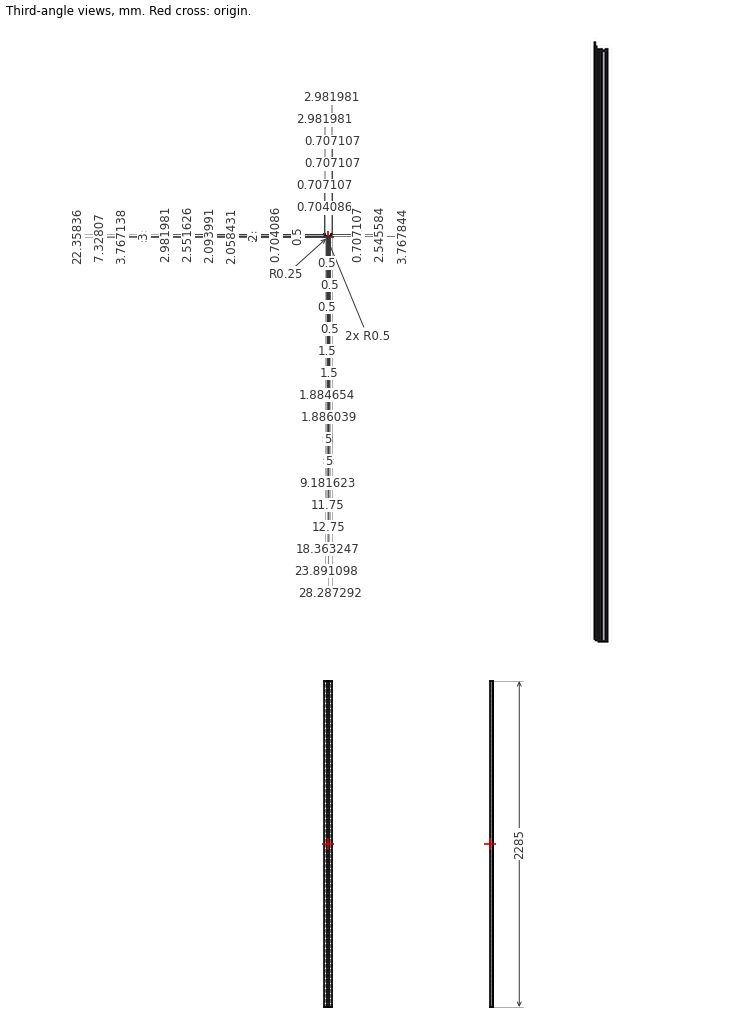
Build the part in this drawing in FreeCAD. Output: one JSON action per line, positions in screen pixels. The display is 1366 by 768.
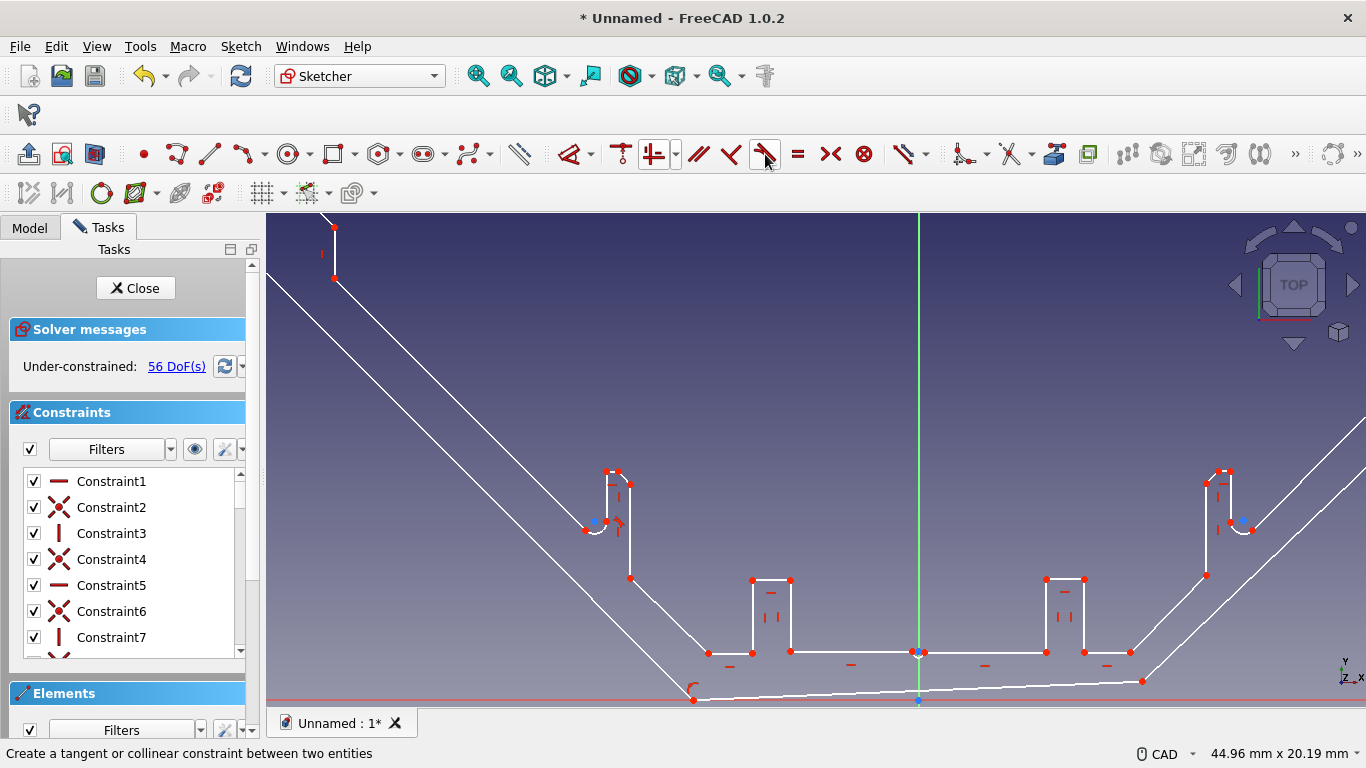
{"action": "left_click", "coordinate": [511, 455]}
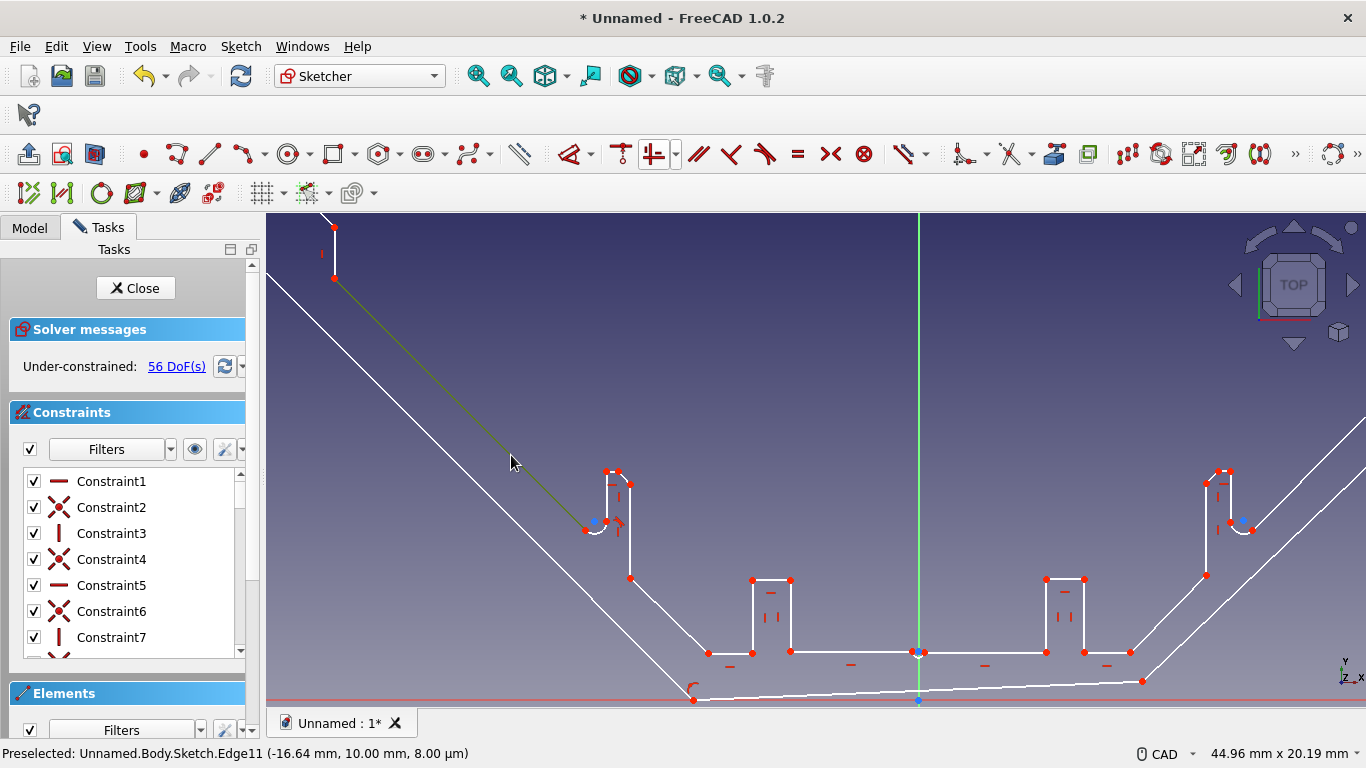
{"action": "left_click", "coordinate": [599, 533]}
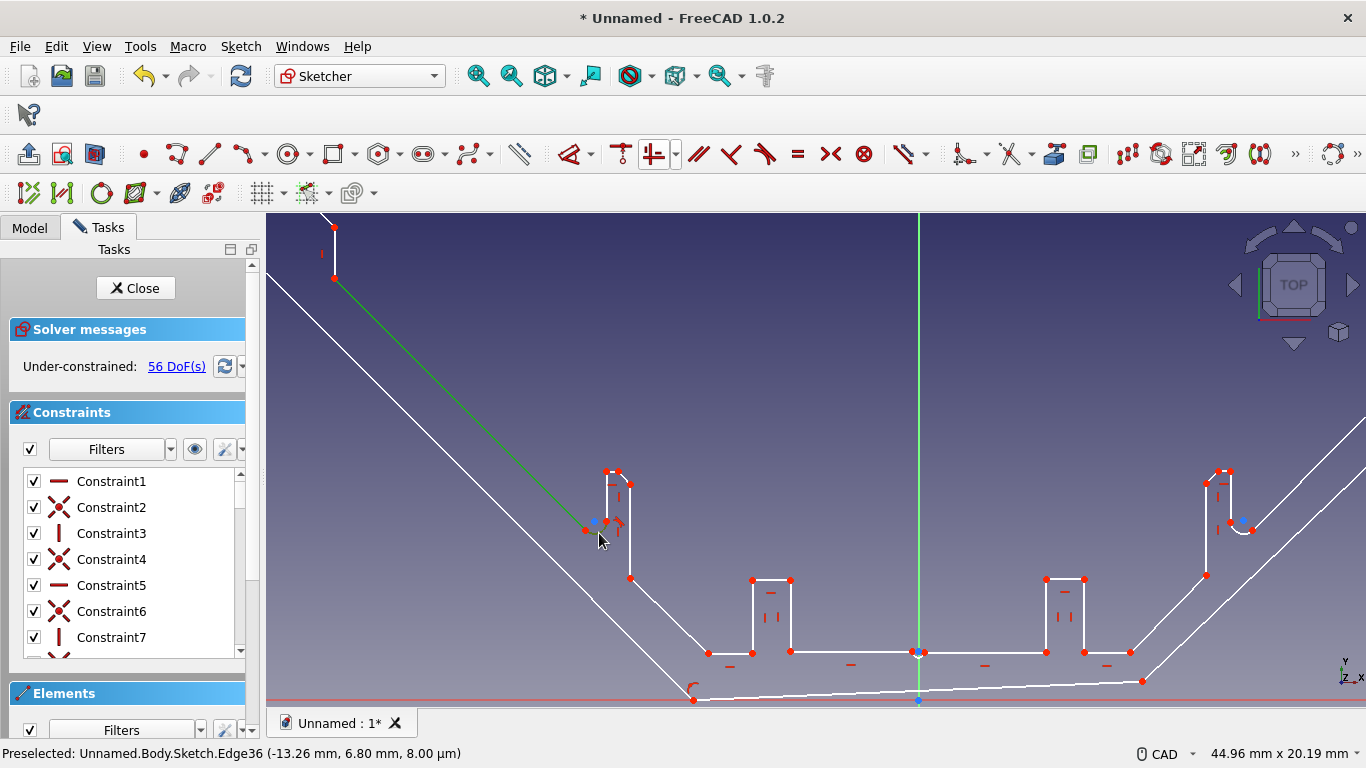
{"action": "left_click", "coordinate": [765, 154]}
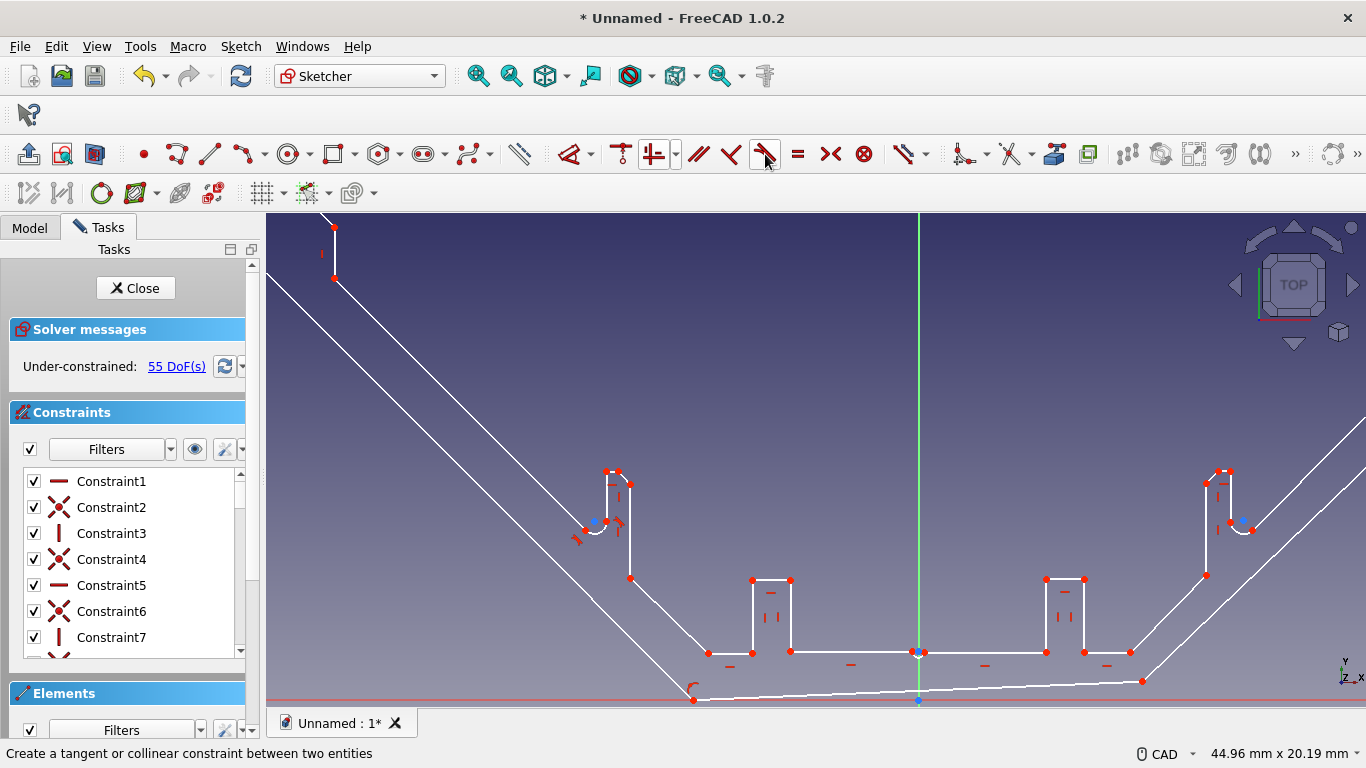
{"action": "scroll", "coordinate": [608, 487], "scroll_direction": "down", "scroll_amount": 4}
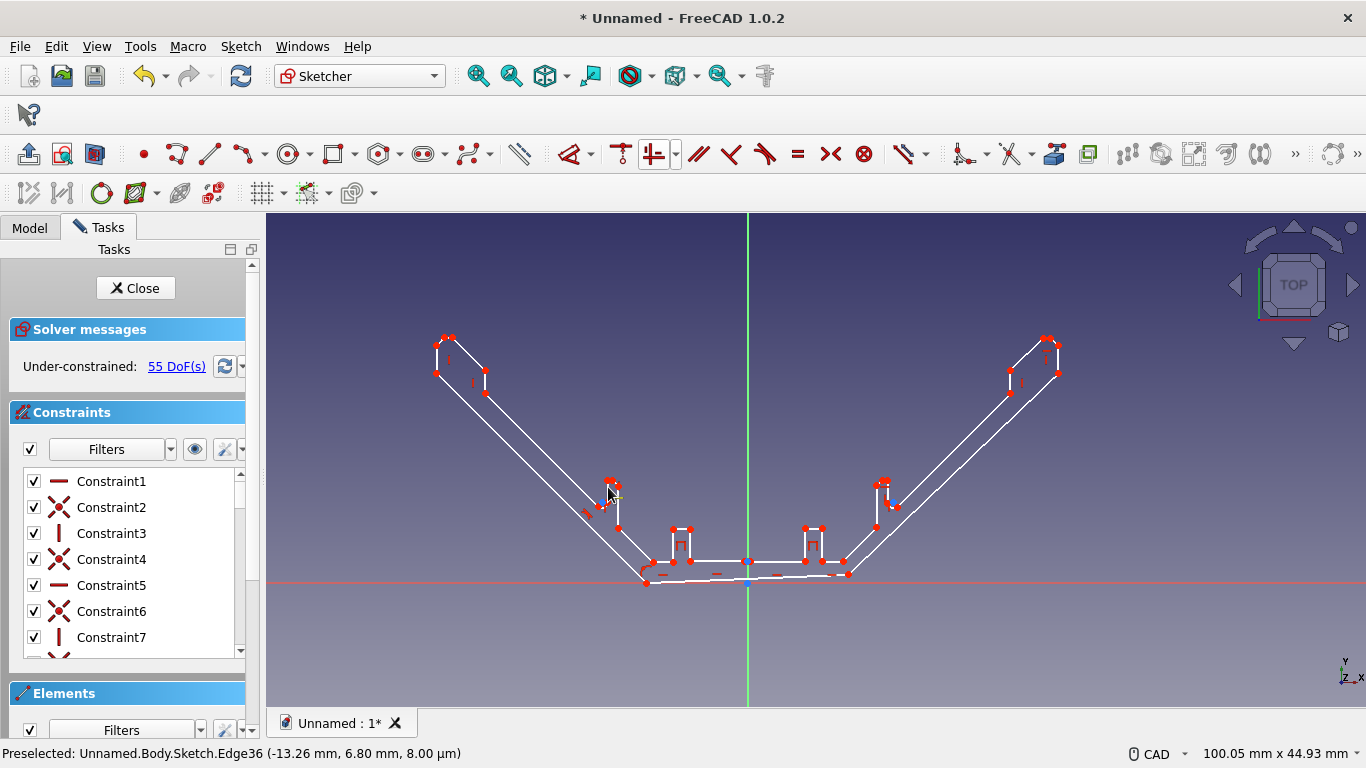
{"action": "left_click", "coordinate": [977, 428]}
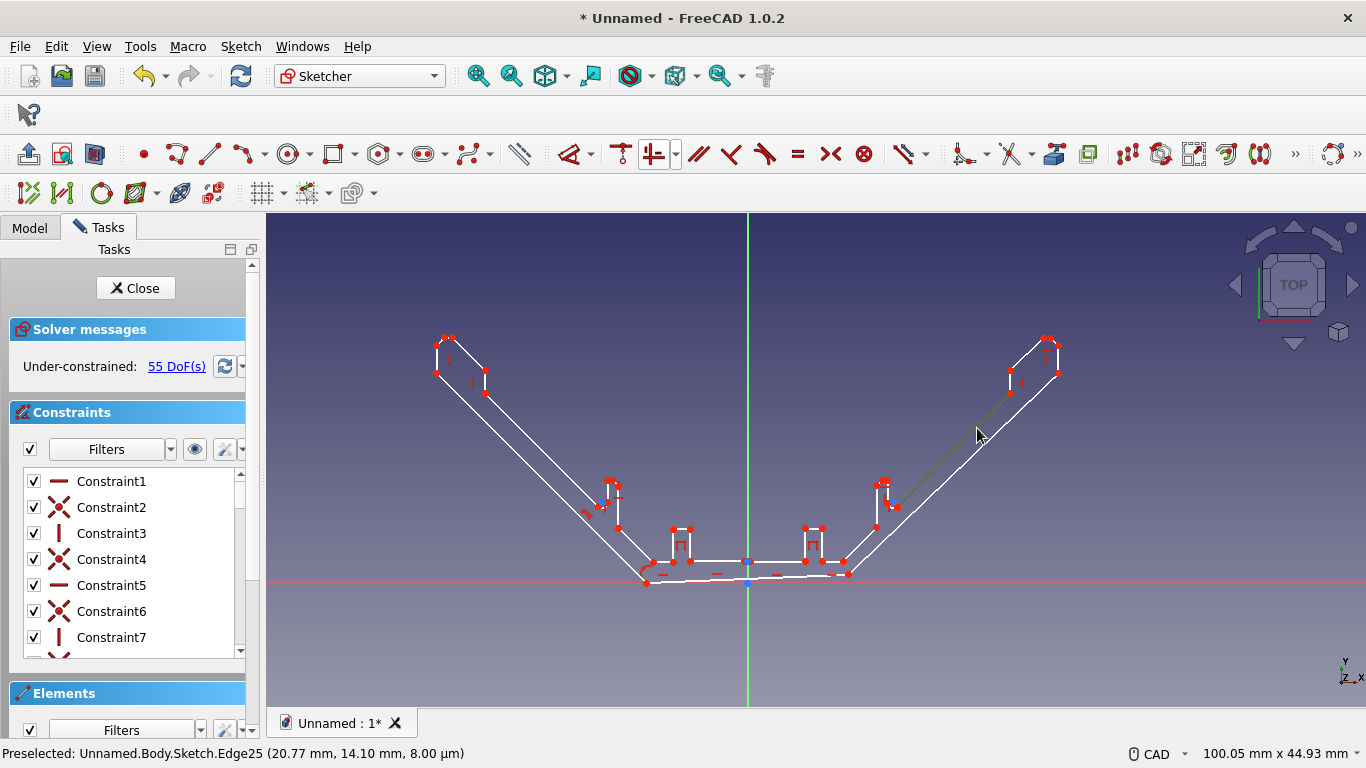
{"action": "scroll", "coordinate": [892, 508], "scroll_direction": "up", "scroll_amount": 5}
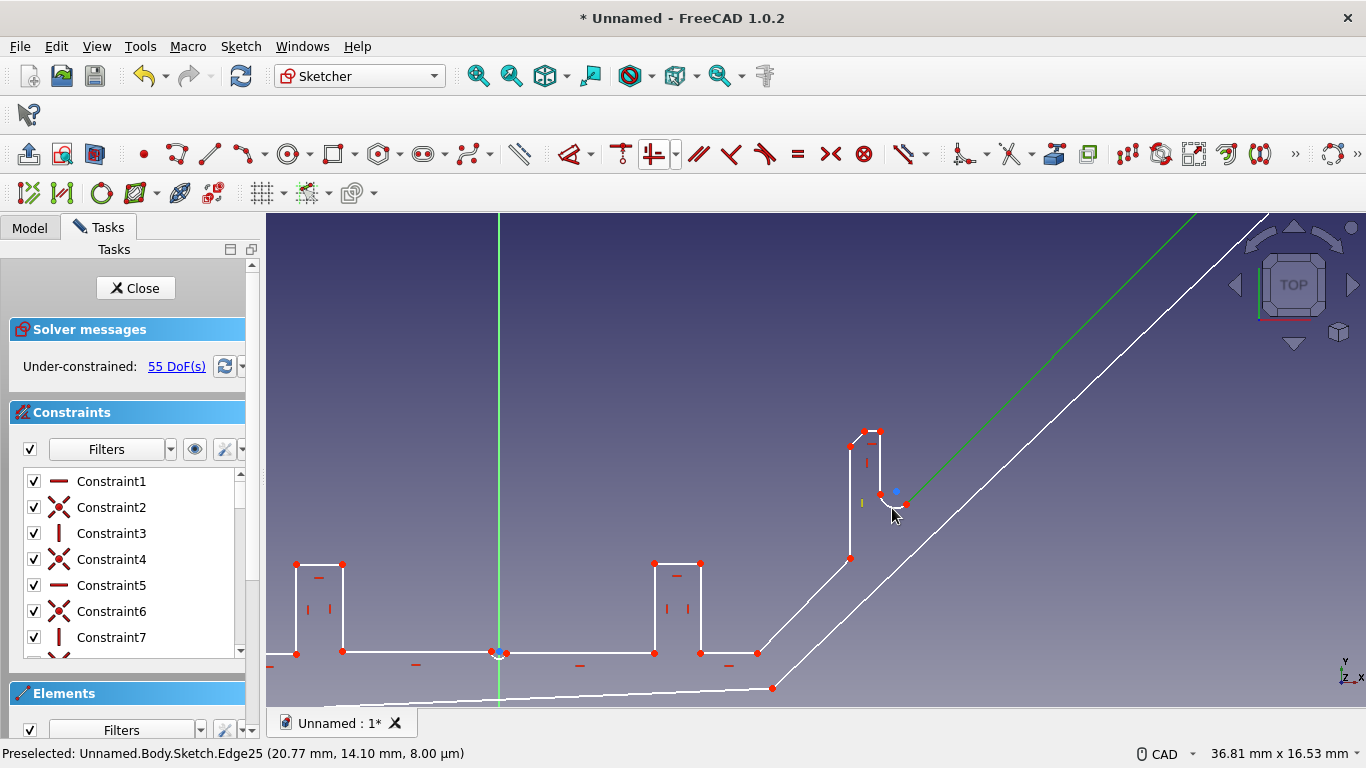
{"action": "left_click", "coordinate": [890, 507]}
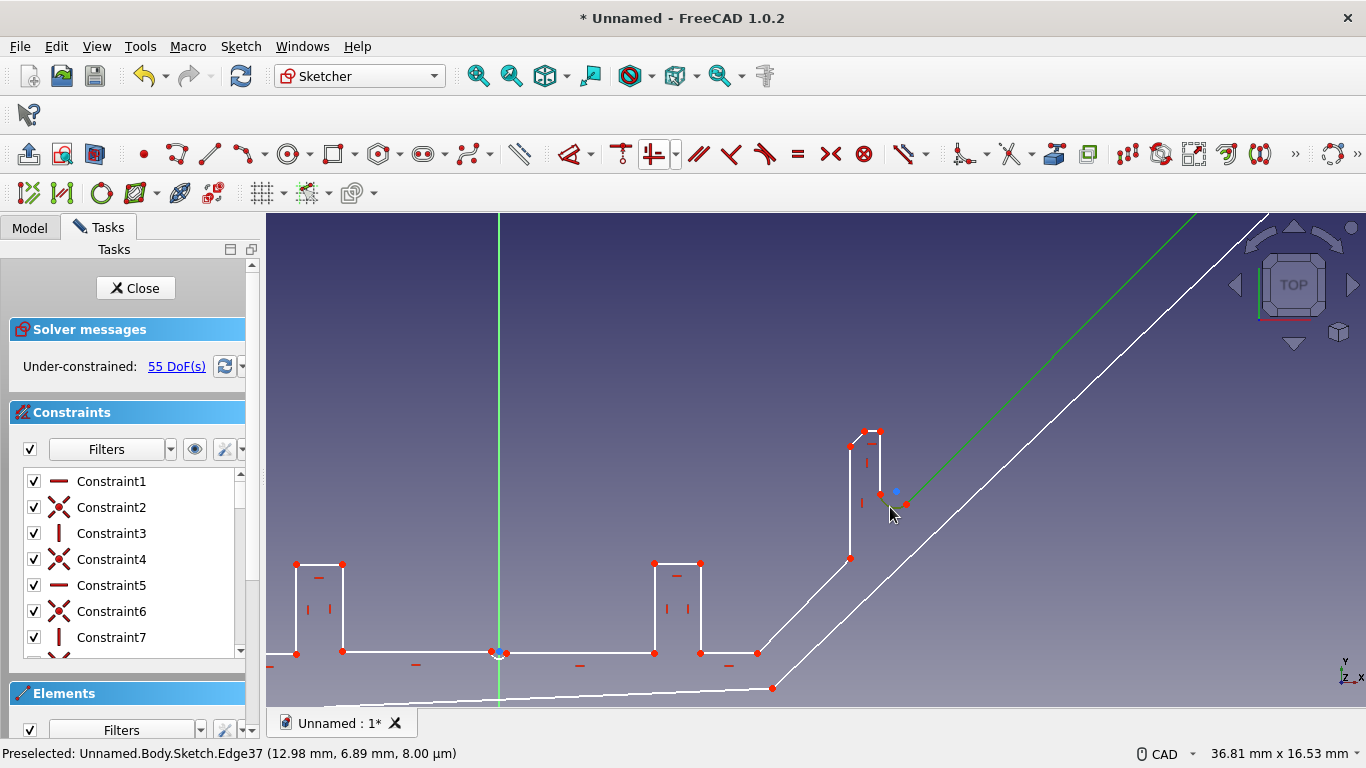
{"action": "left_click", "coordinate": [765, 154]}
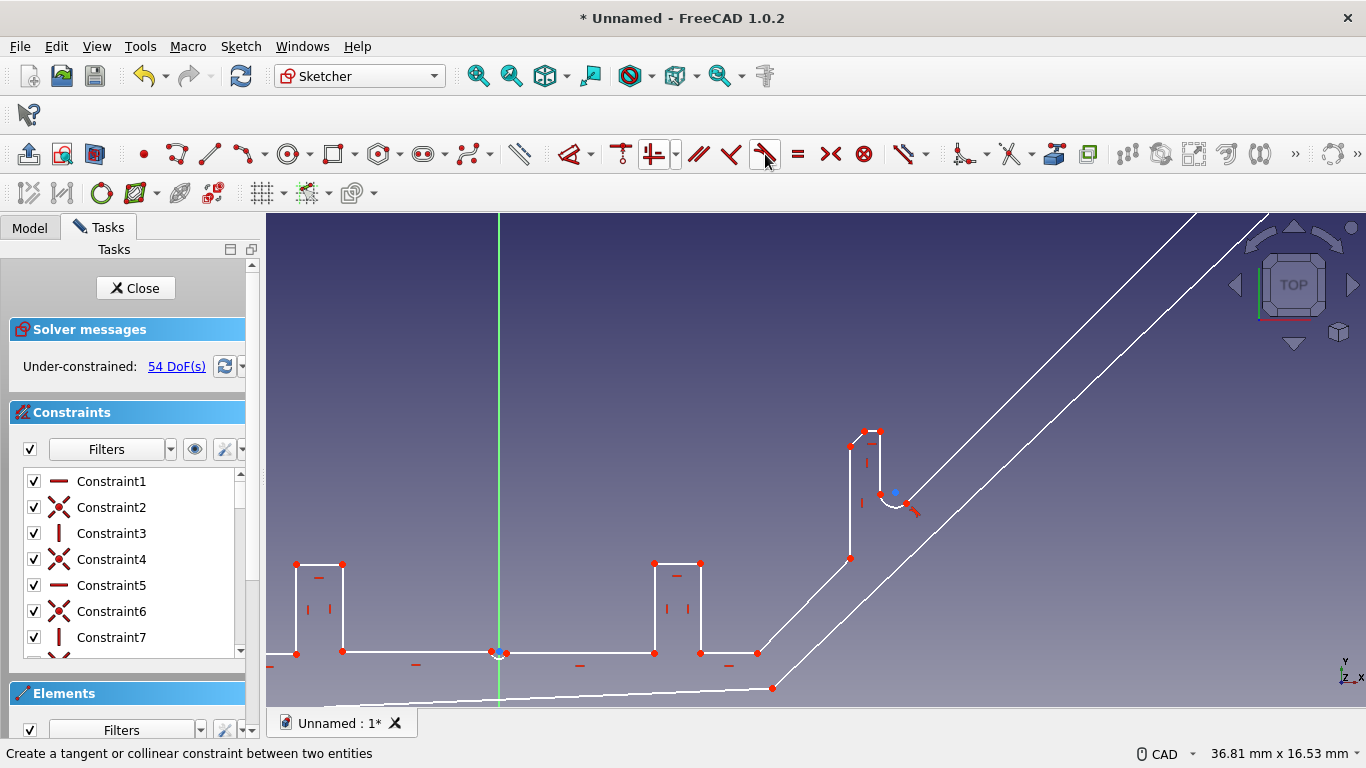
{"action": "left_click", "coordinate": [880, 475]}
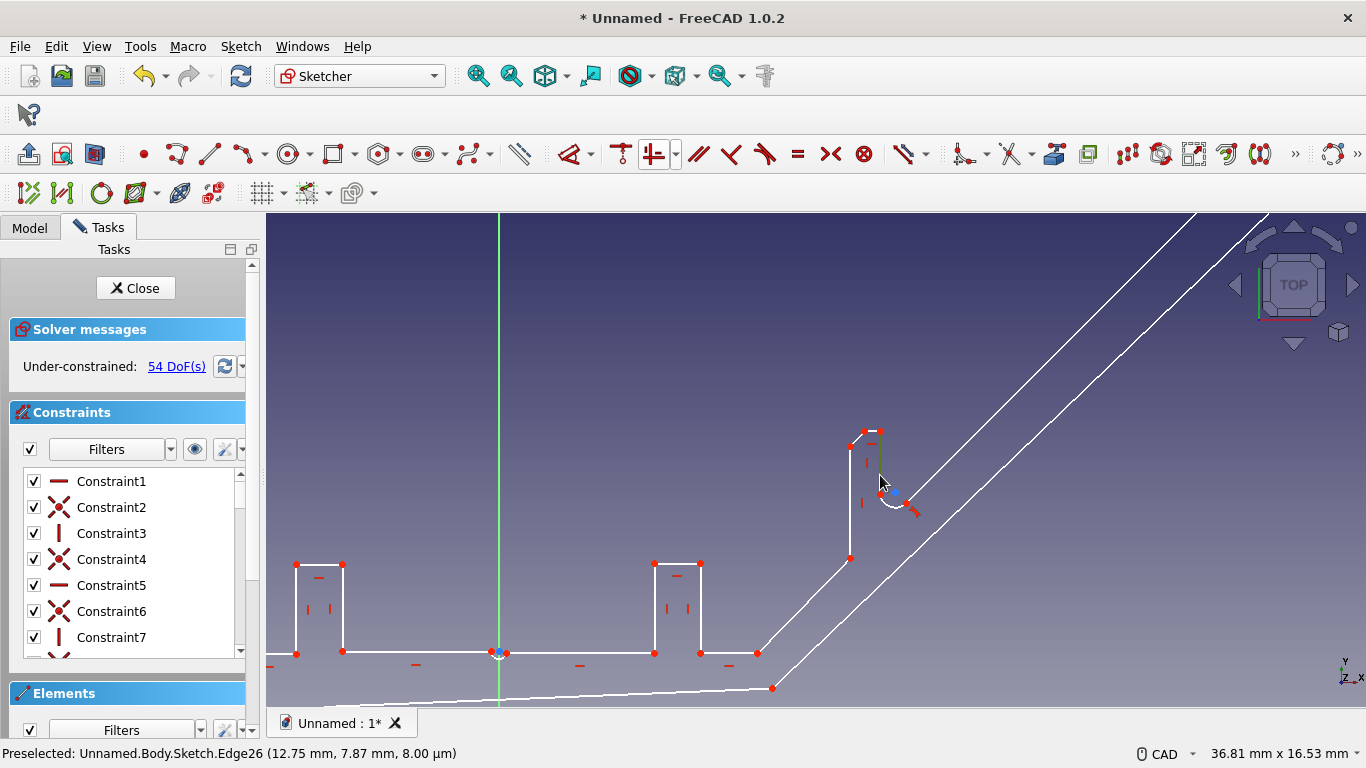
{"action": "scroll", "coordinate": [885, 503], "scroll_direction": "up", "scroll_amount": 2}